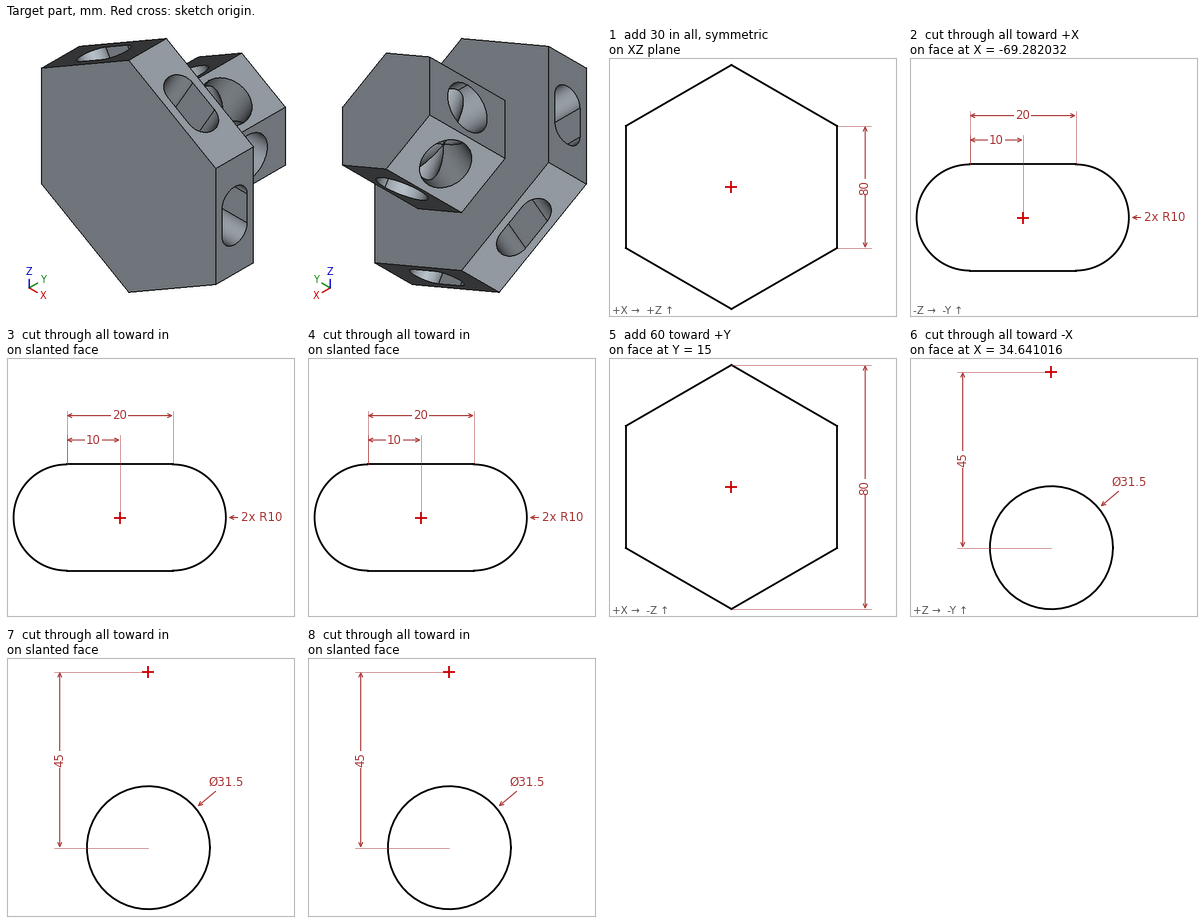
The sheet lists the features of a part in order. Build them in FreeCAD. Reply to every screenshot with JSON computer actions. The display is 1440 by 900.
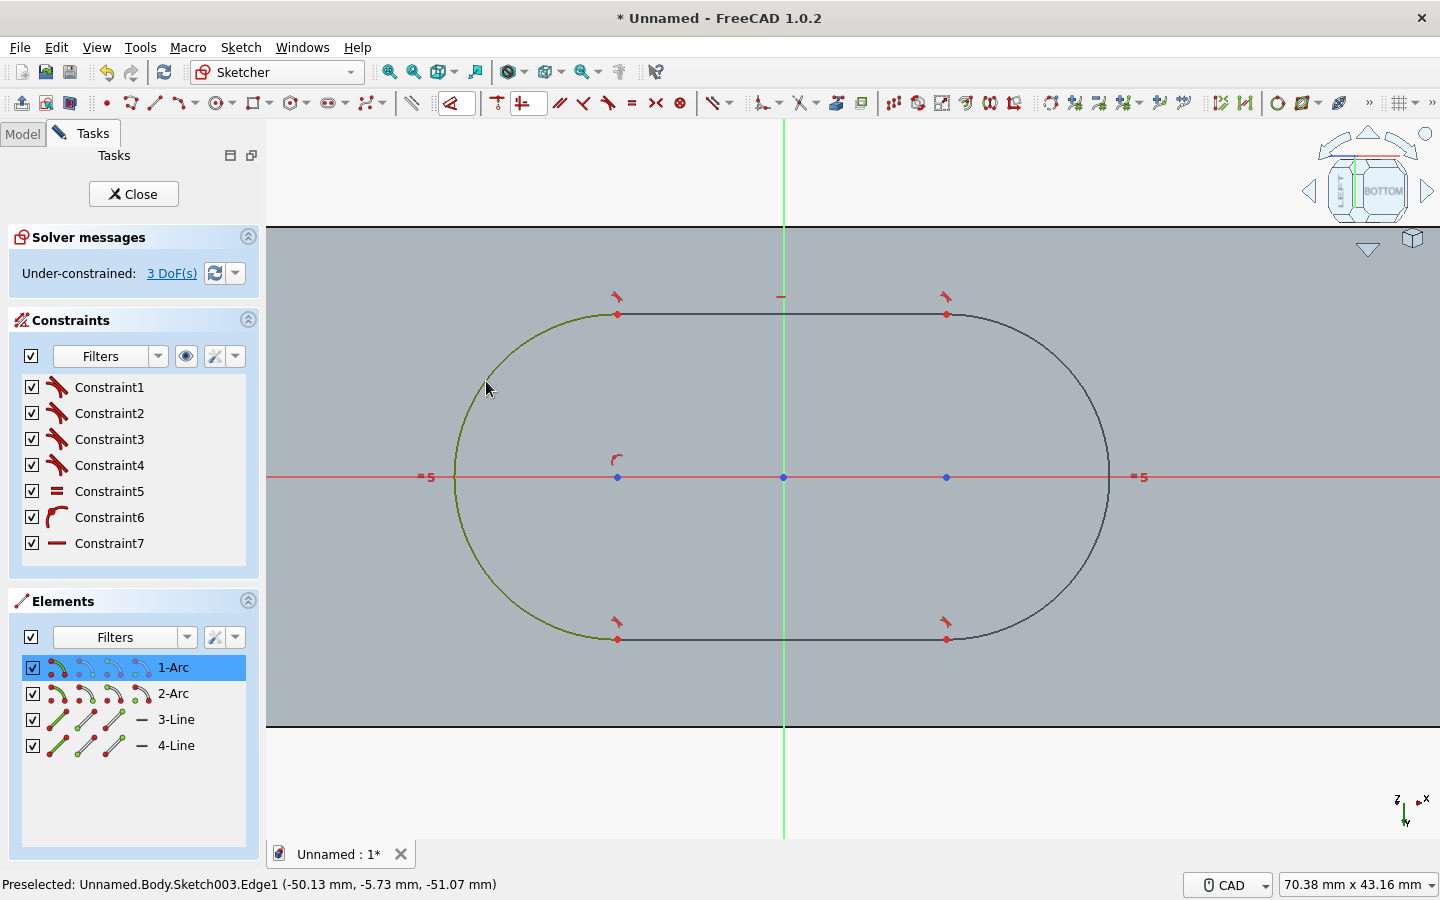
{"action": "left_click", "coordinate": [470, 104]}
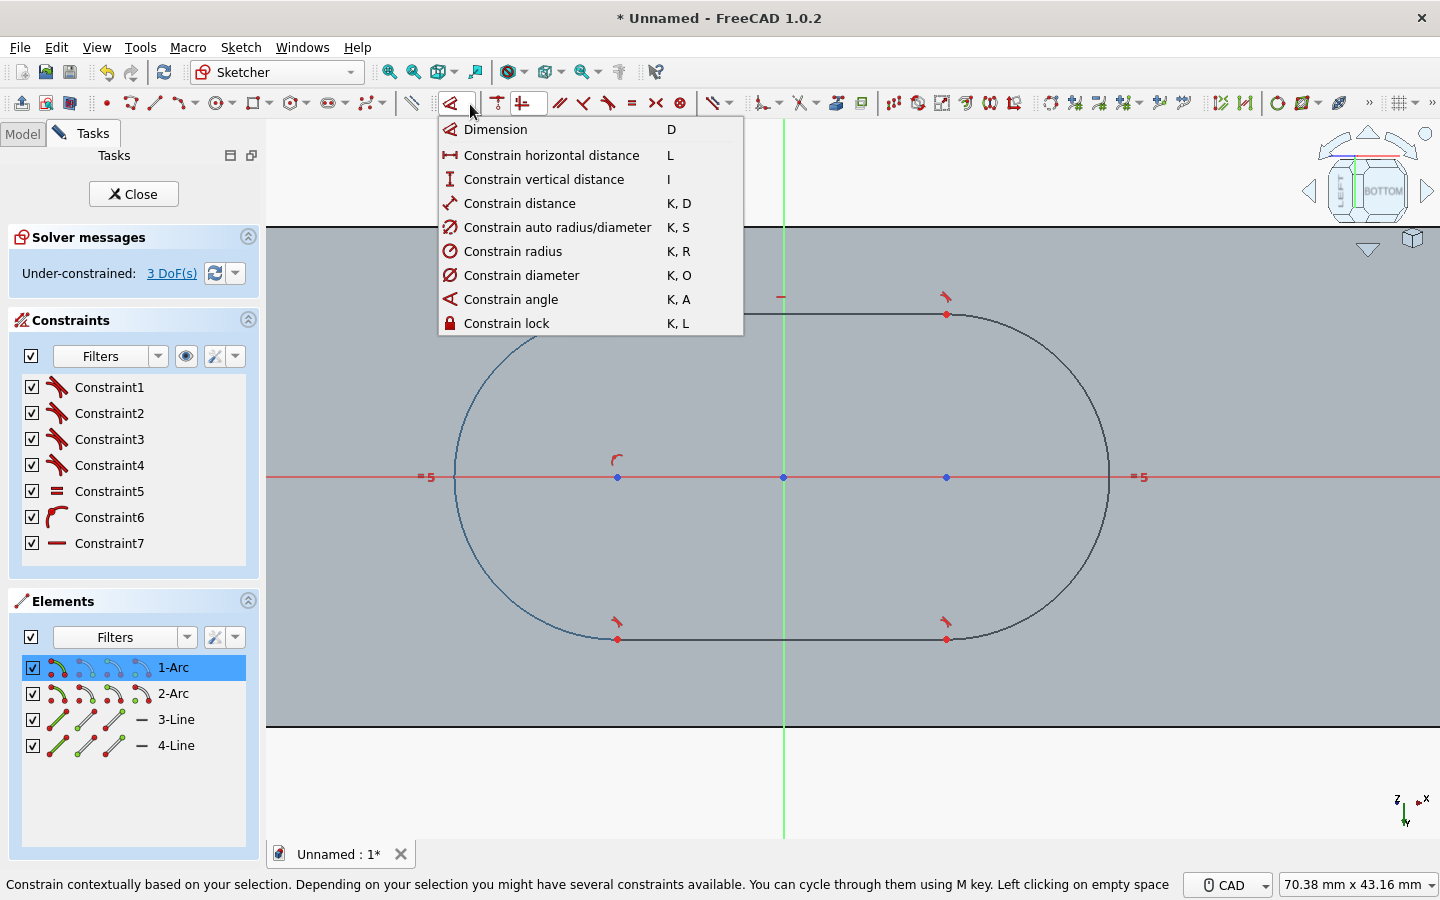
{"action": "left_click", "coordinate": [591, 251]}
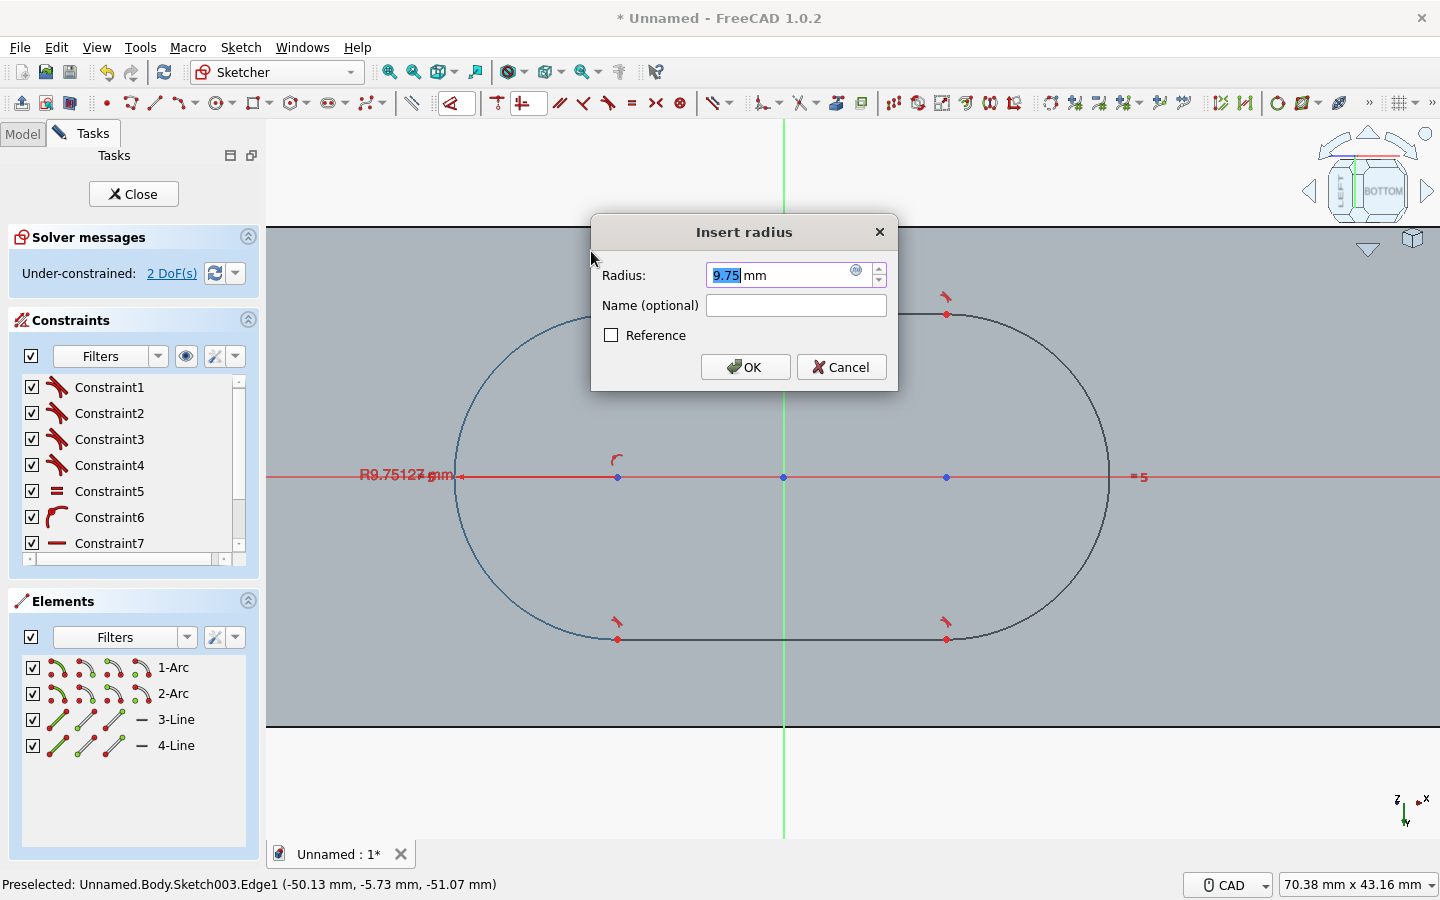
{"action": "type", "text": "10"}
{"action": "key", "text": "Return"}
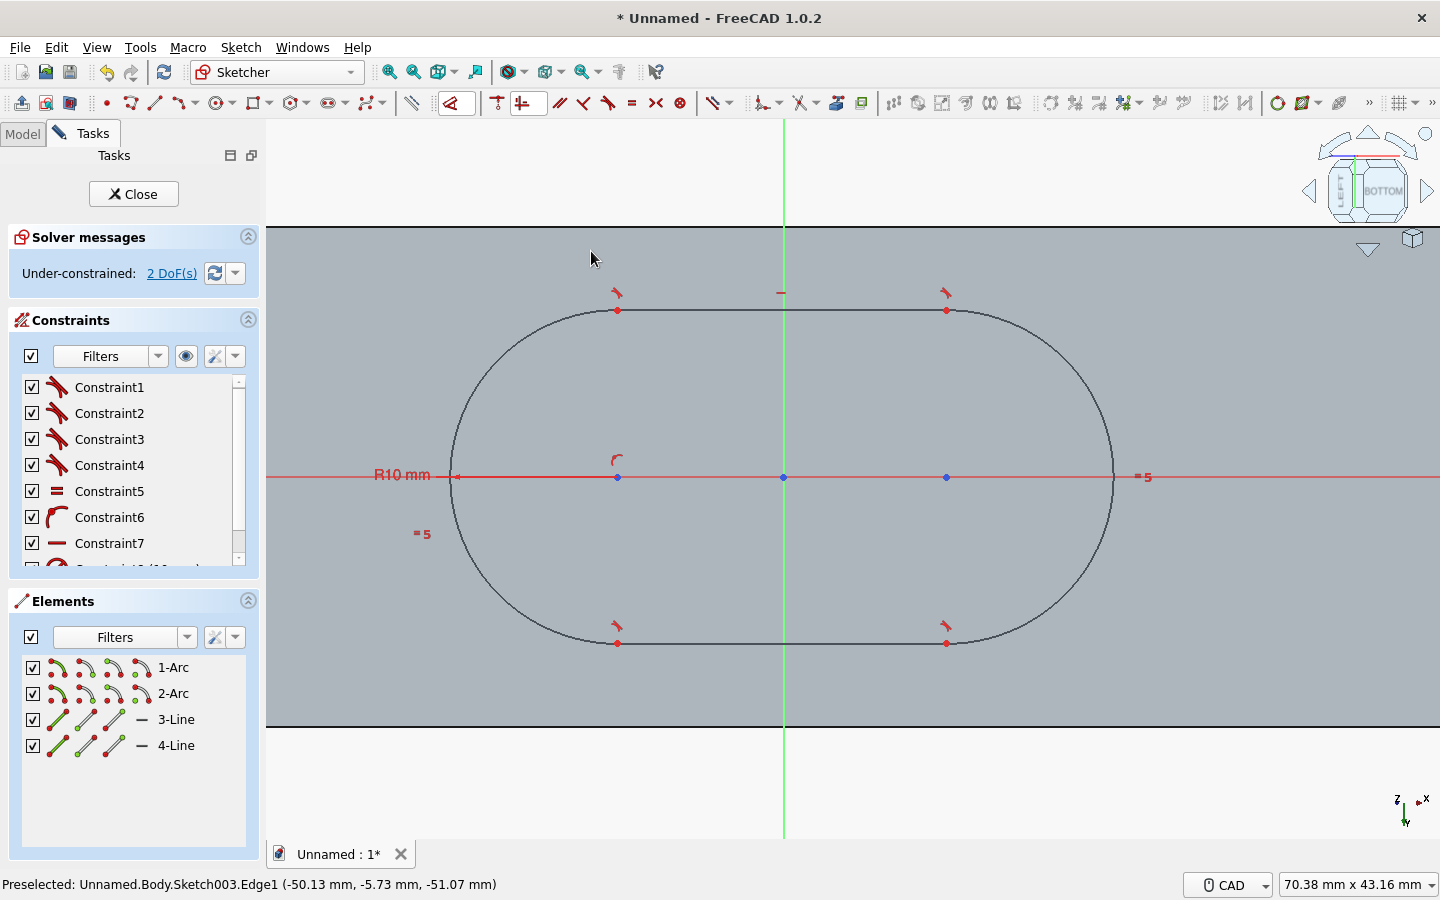
{"action": "left_click", "coordinate": [716, 310]}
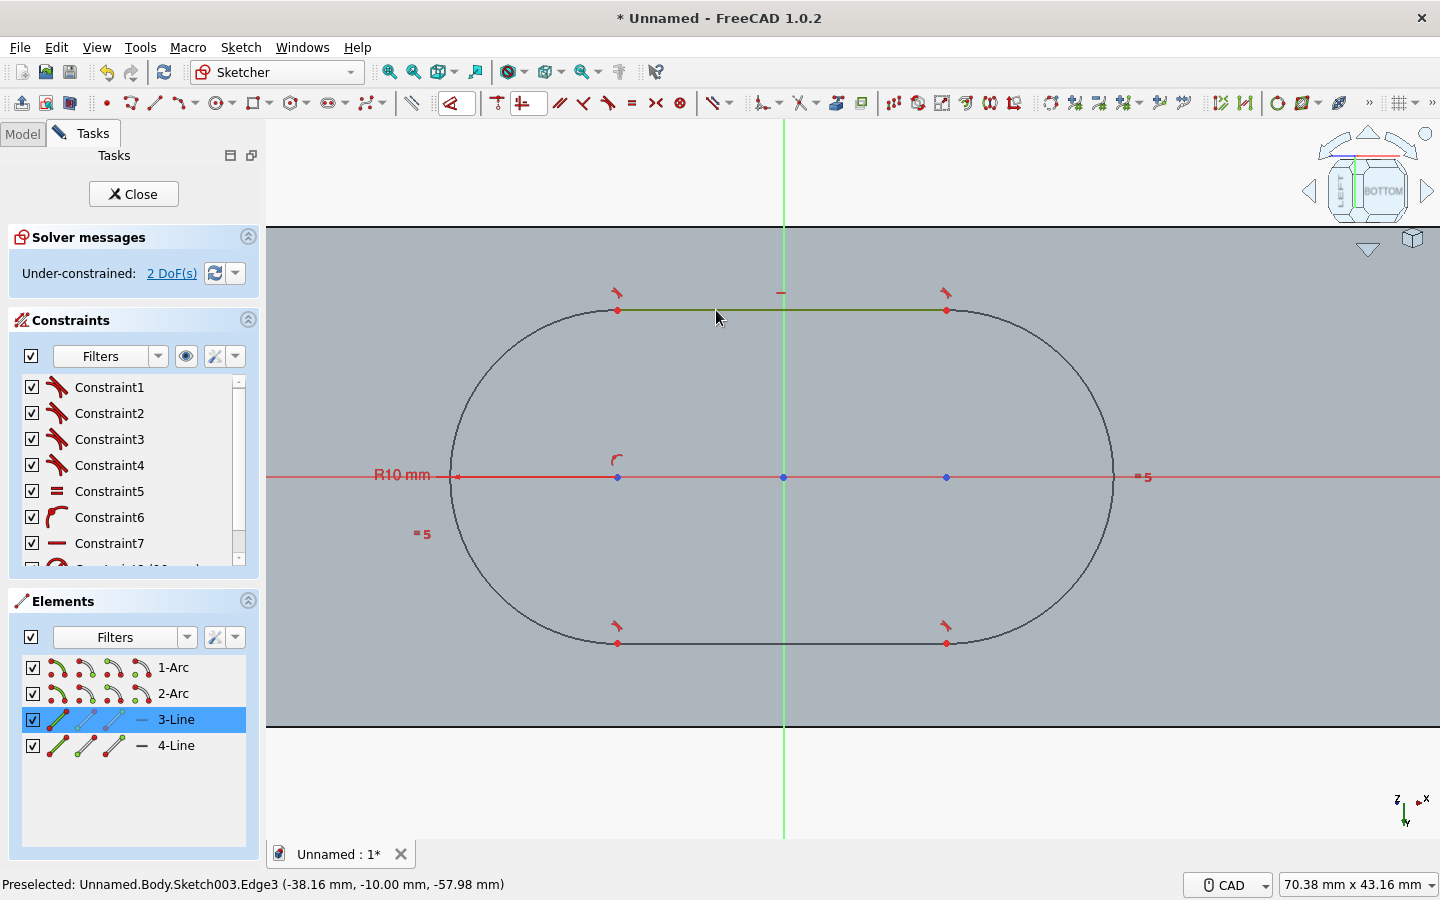
{"action": "left_click", "coordinate": [470, 104]}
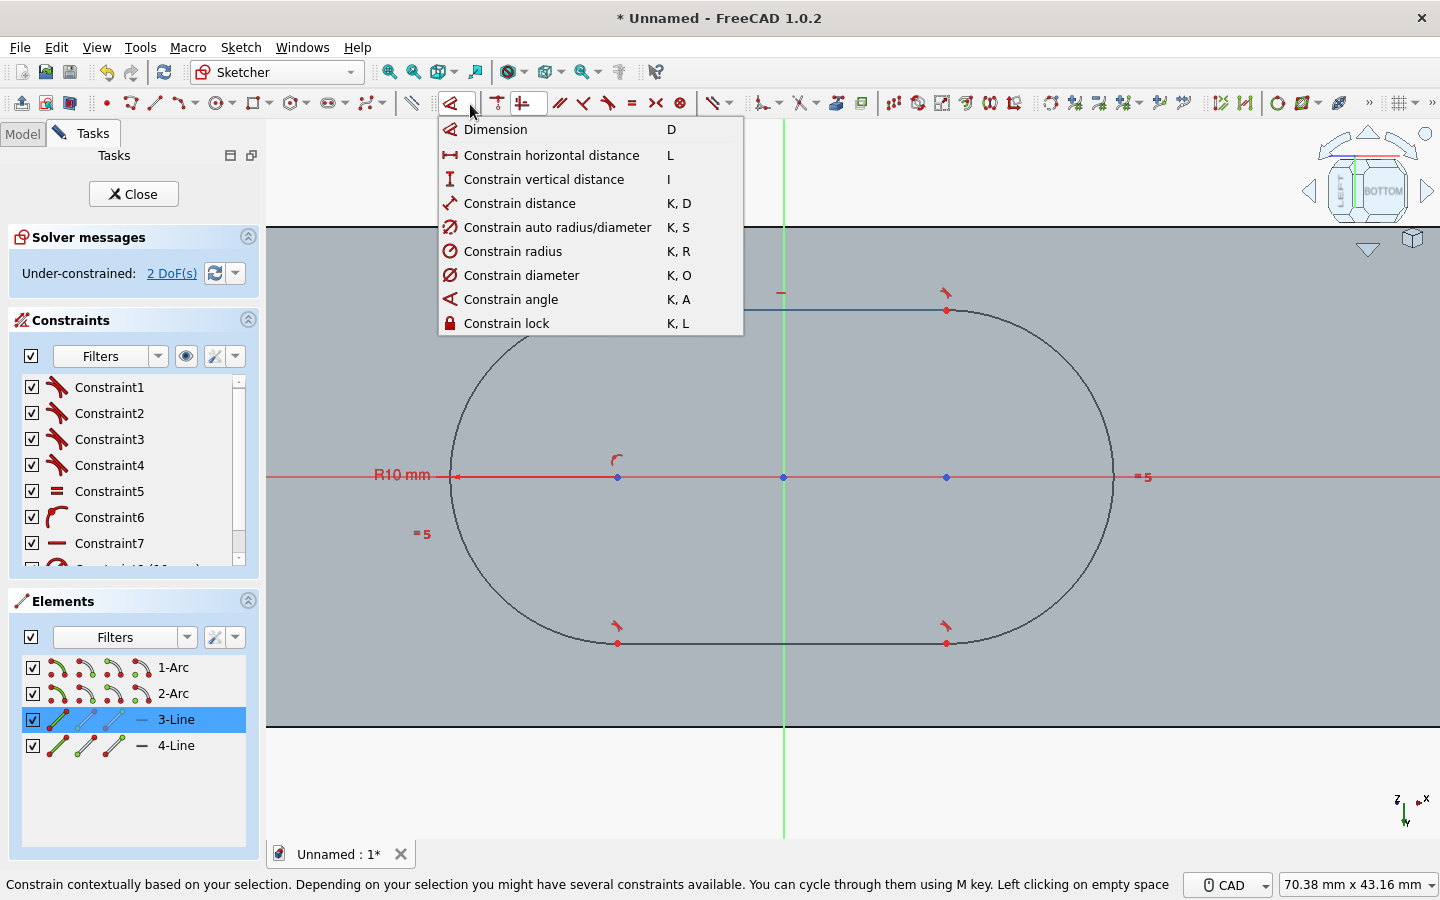
{"action": "left_click", "coordinate": [591, 155]}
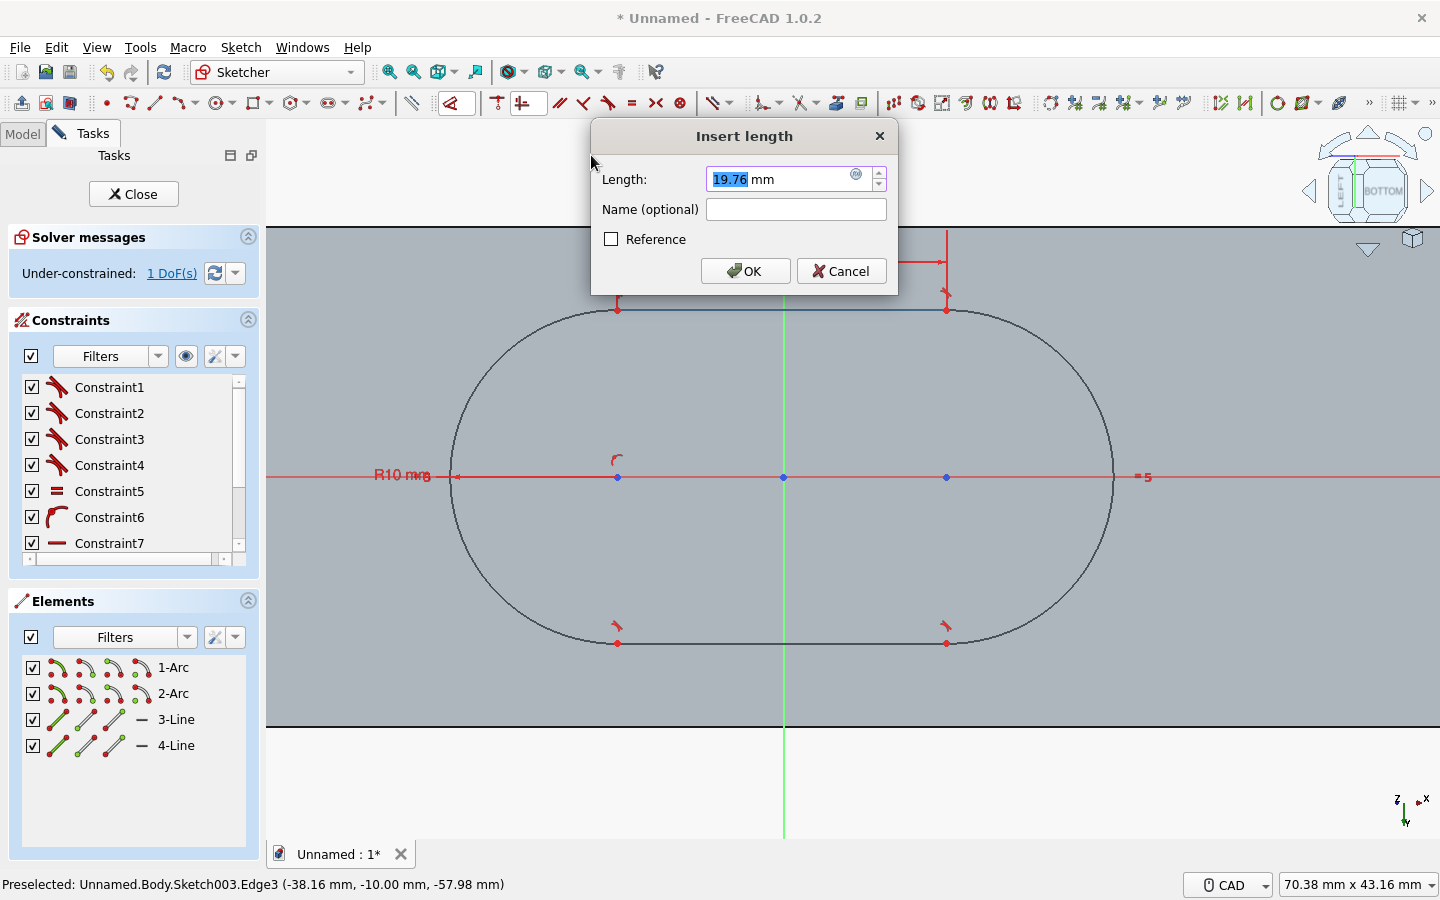
{"action": "type", "text": "20"}
{"action": "key", "text": "Return"}